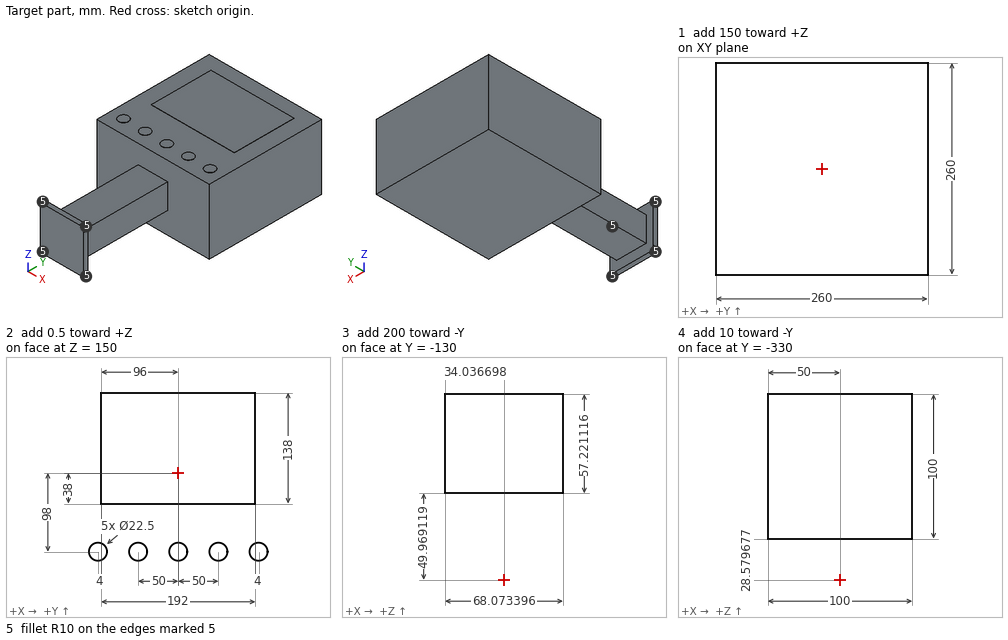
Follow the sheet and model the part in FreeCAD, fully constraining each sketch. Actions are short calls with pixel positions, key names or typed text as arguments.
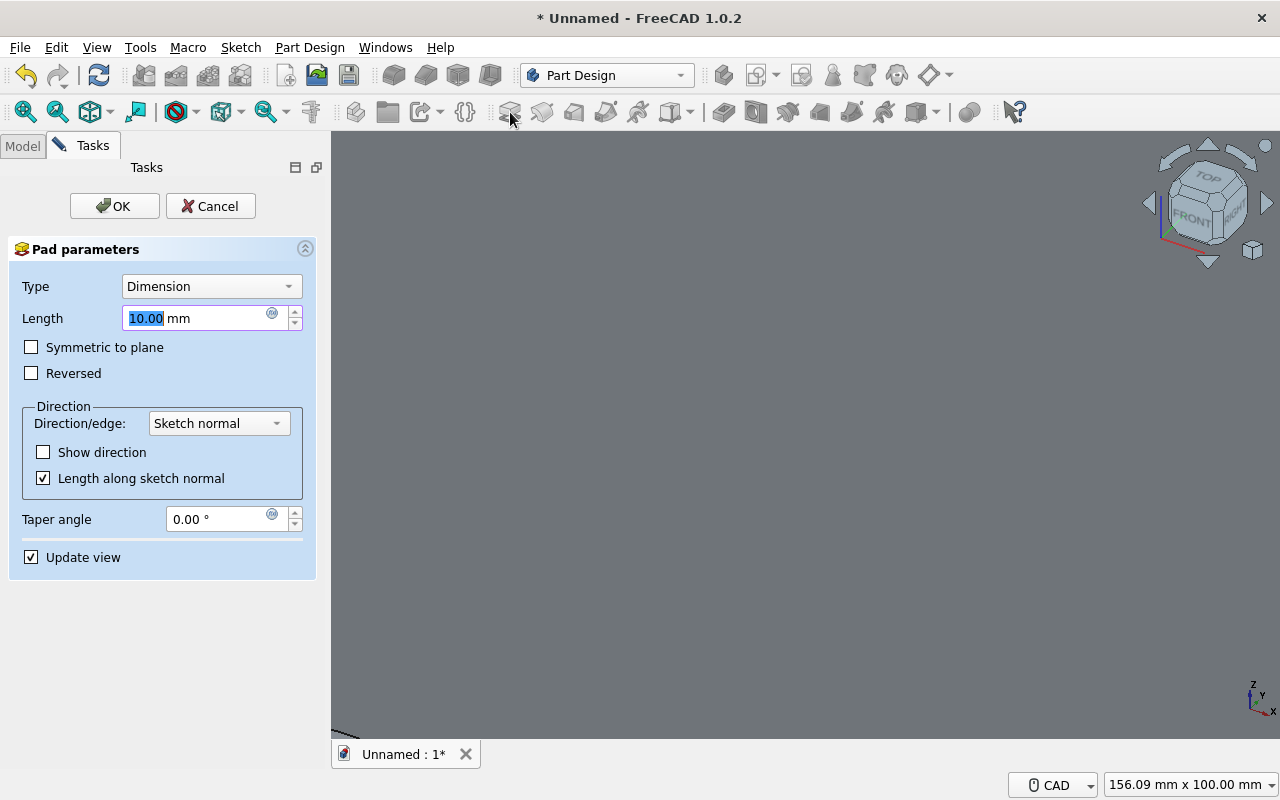
text(150)
key(Tab)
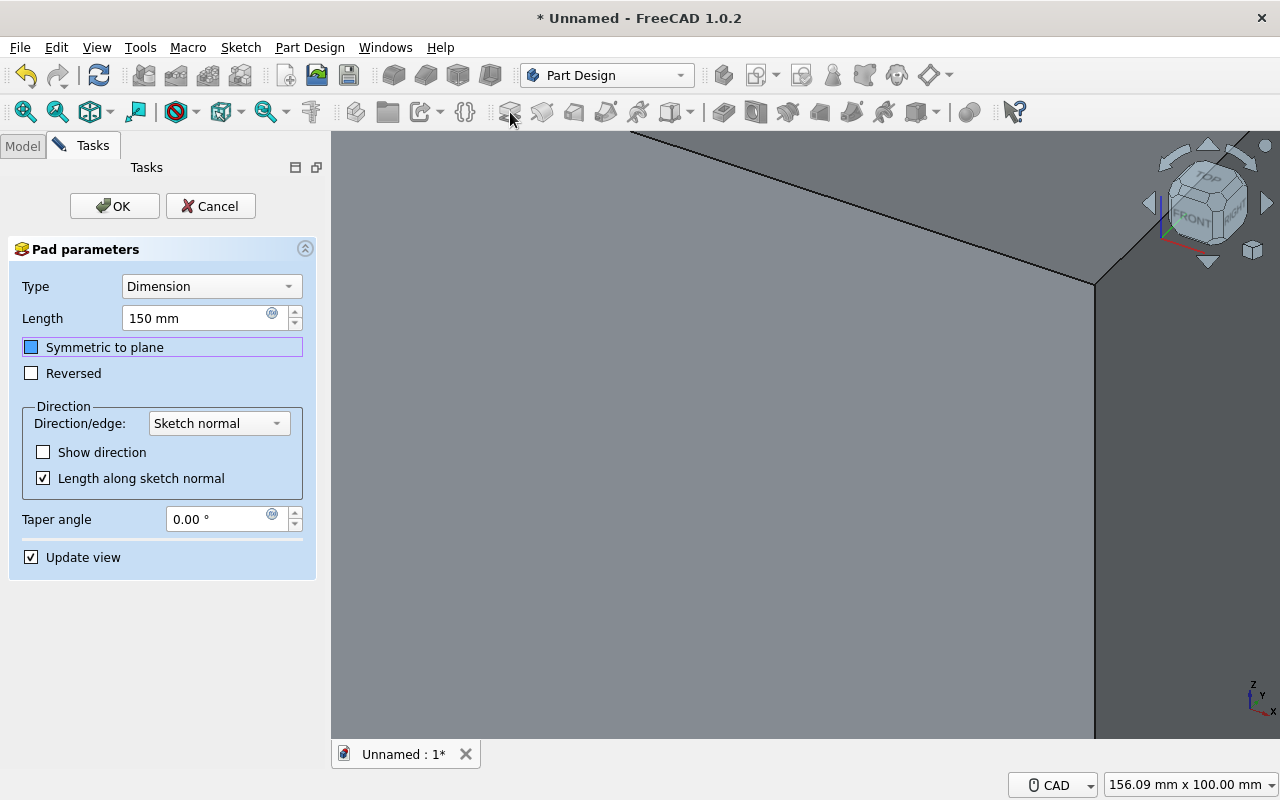
click(115, 206)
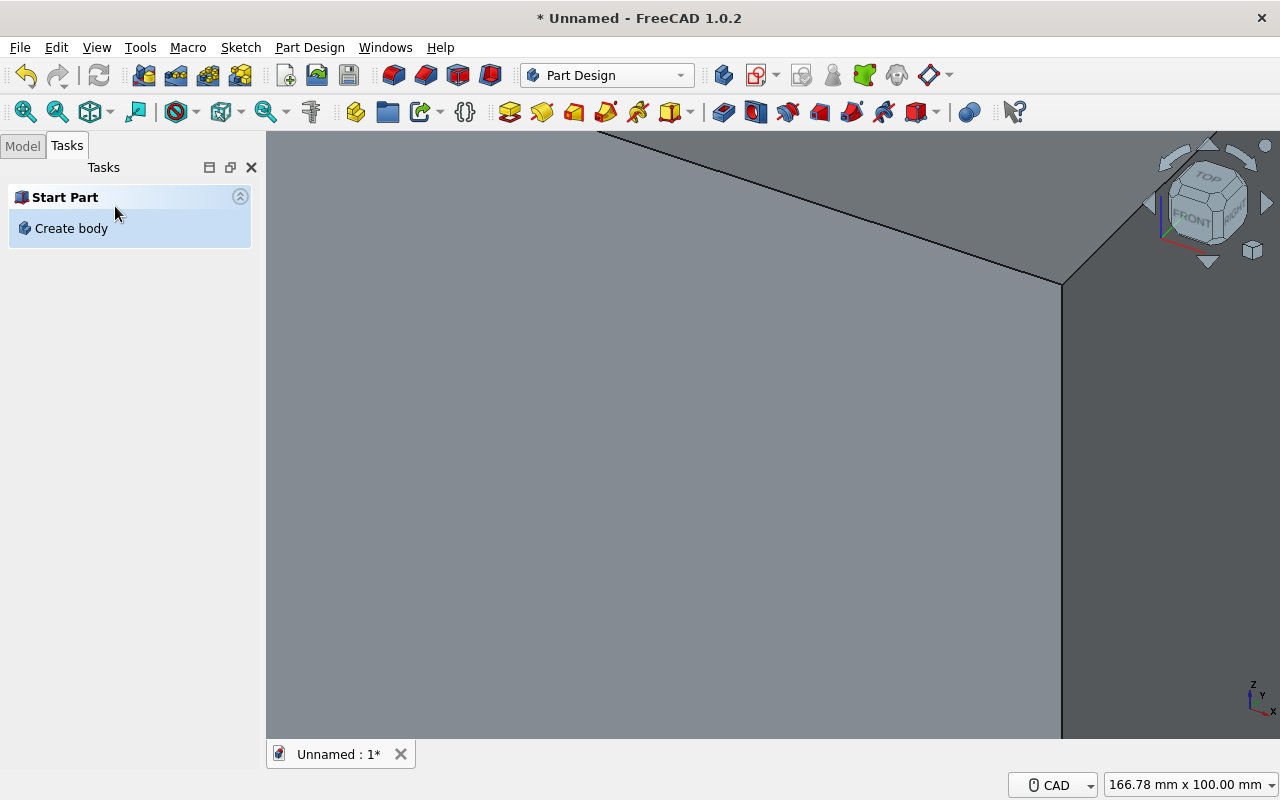
key(v)
key(f)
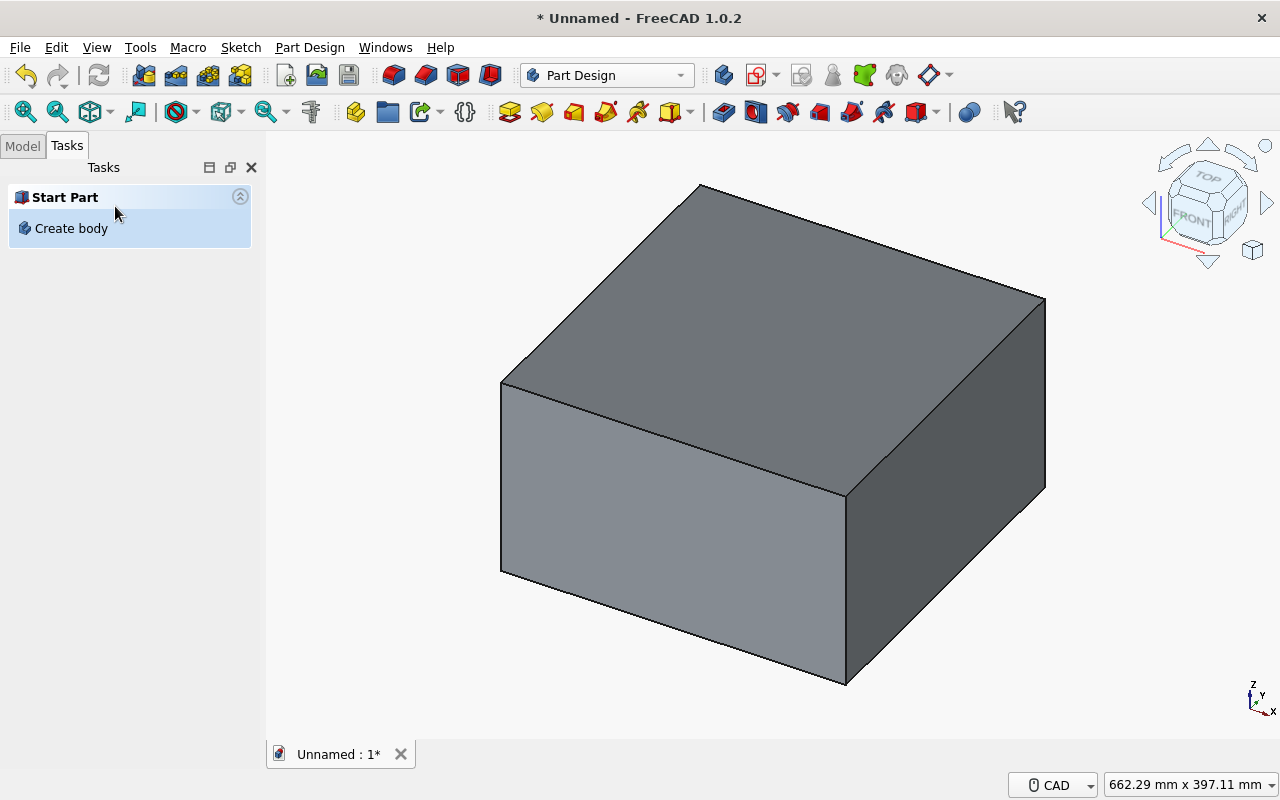
click(773, 340)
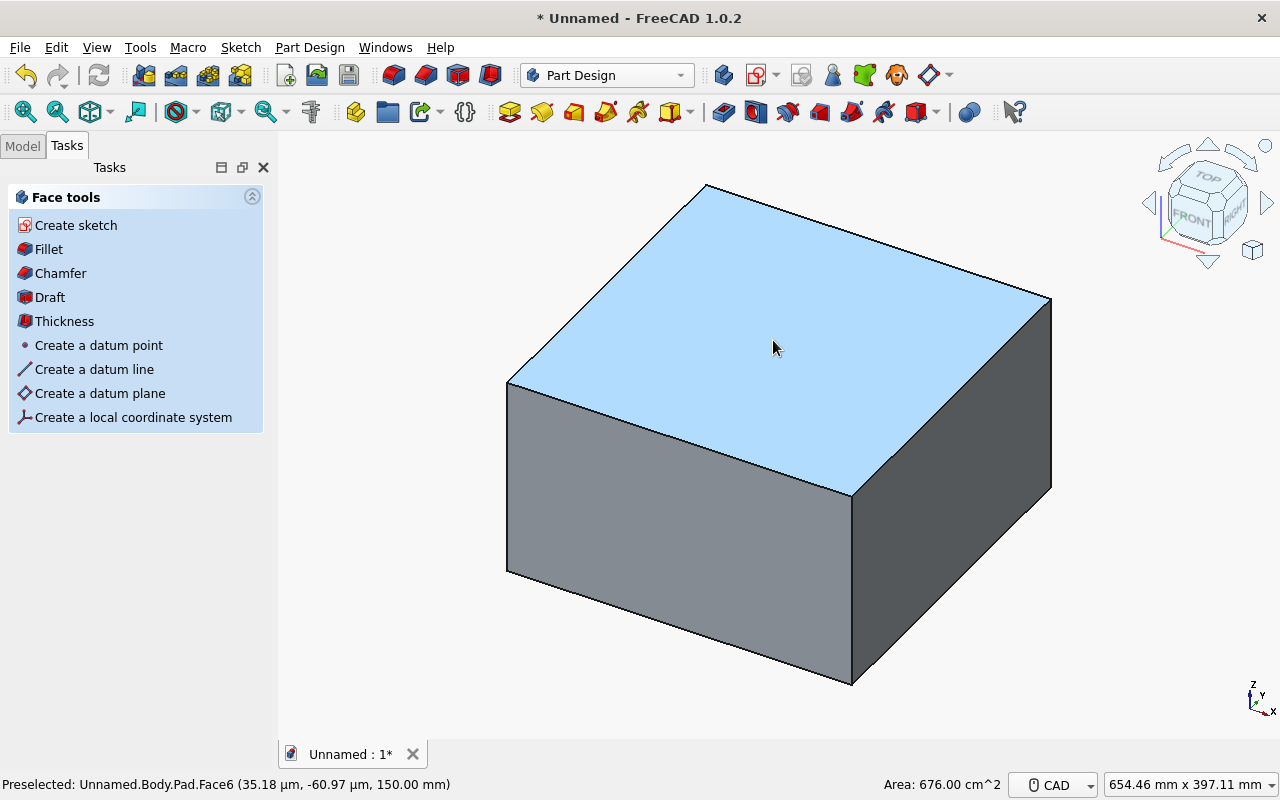
click(756, 76)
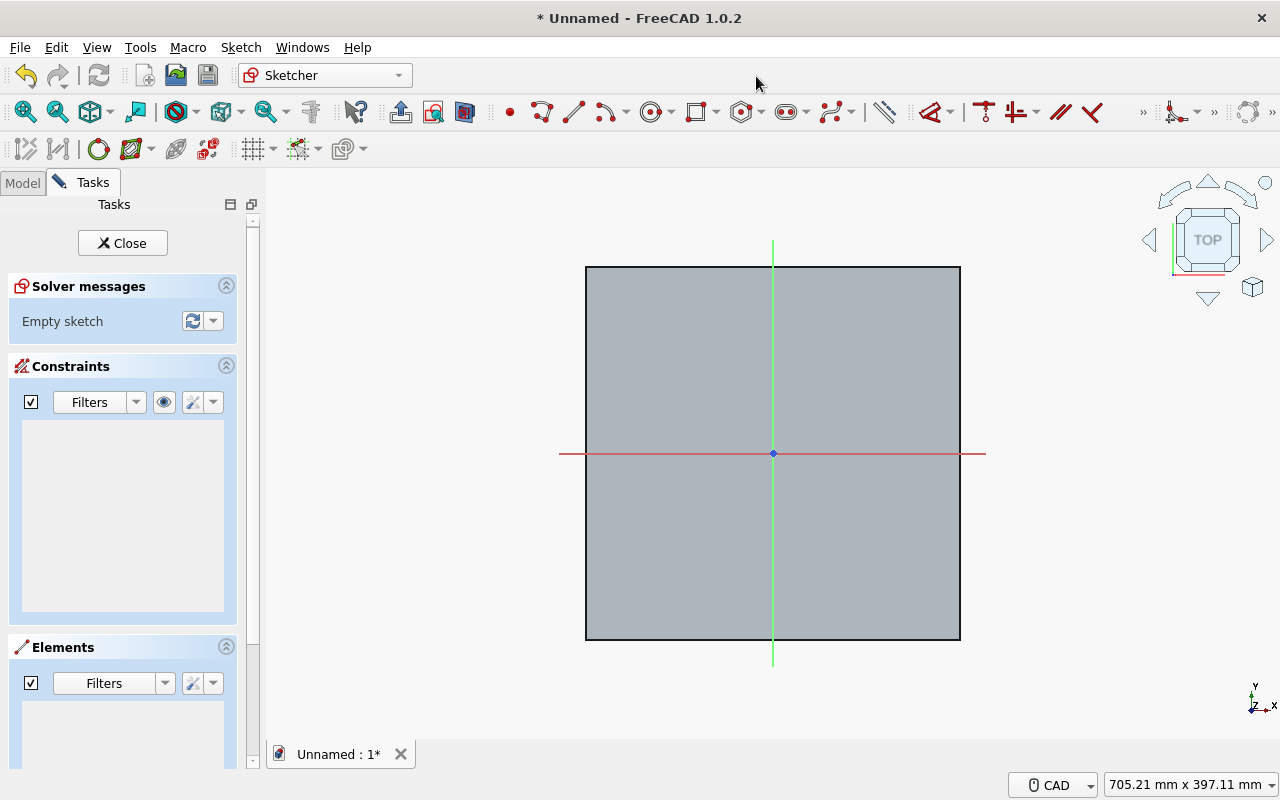
click(696, 112)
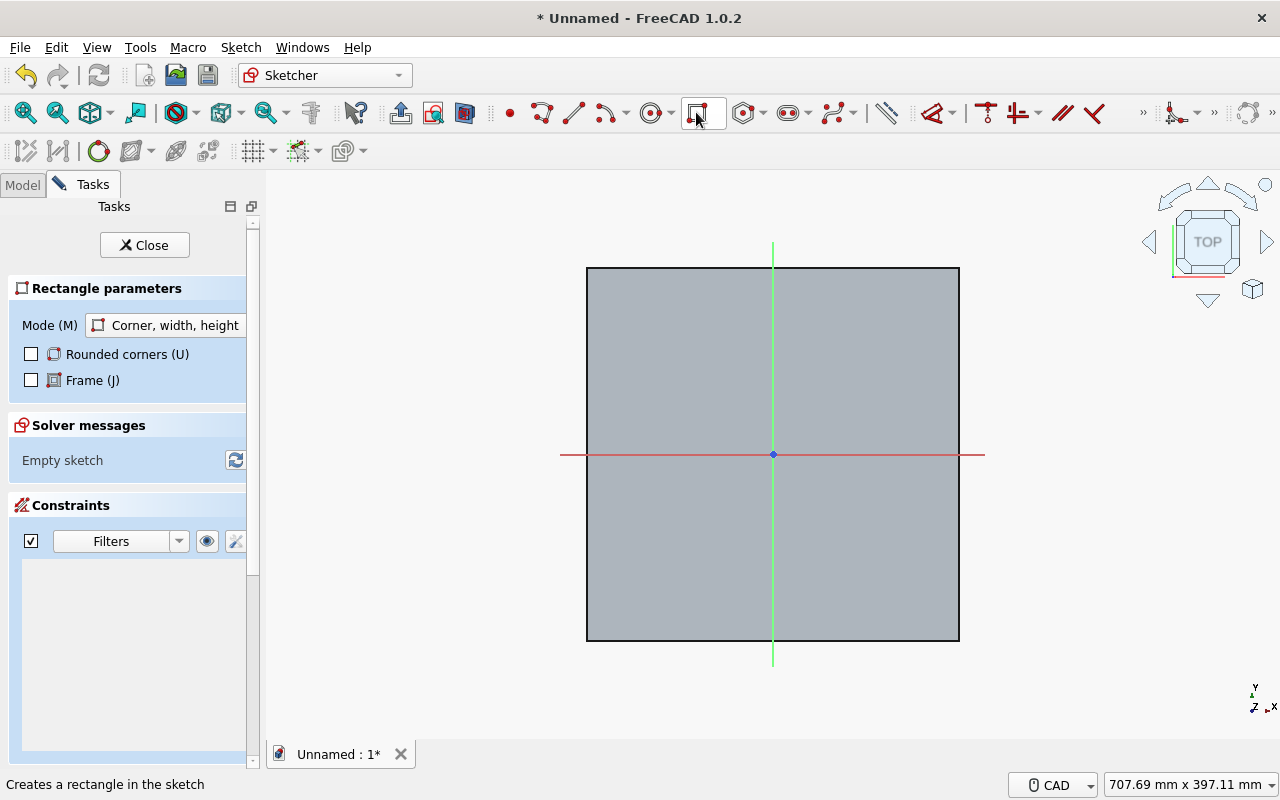
click(635, 311)
move(911, 509)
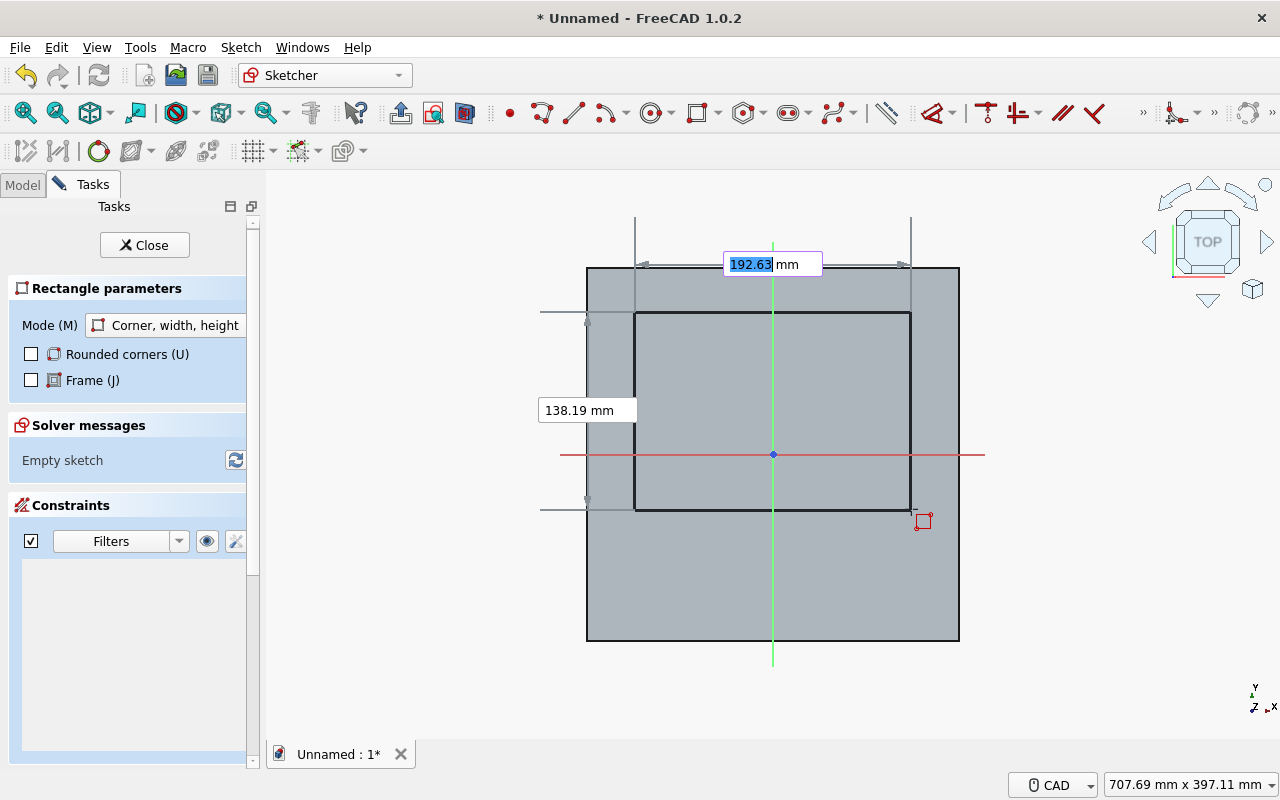
text(192)
key(Tab)
text(138)
key(Return)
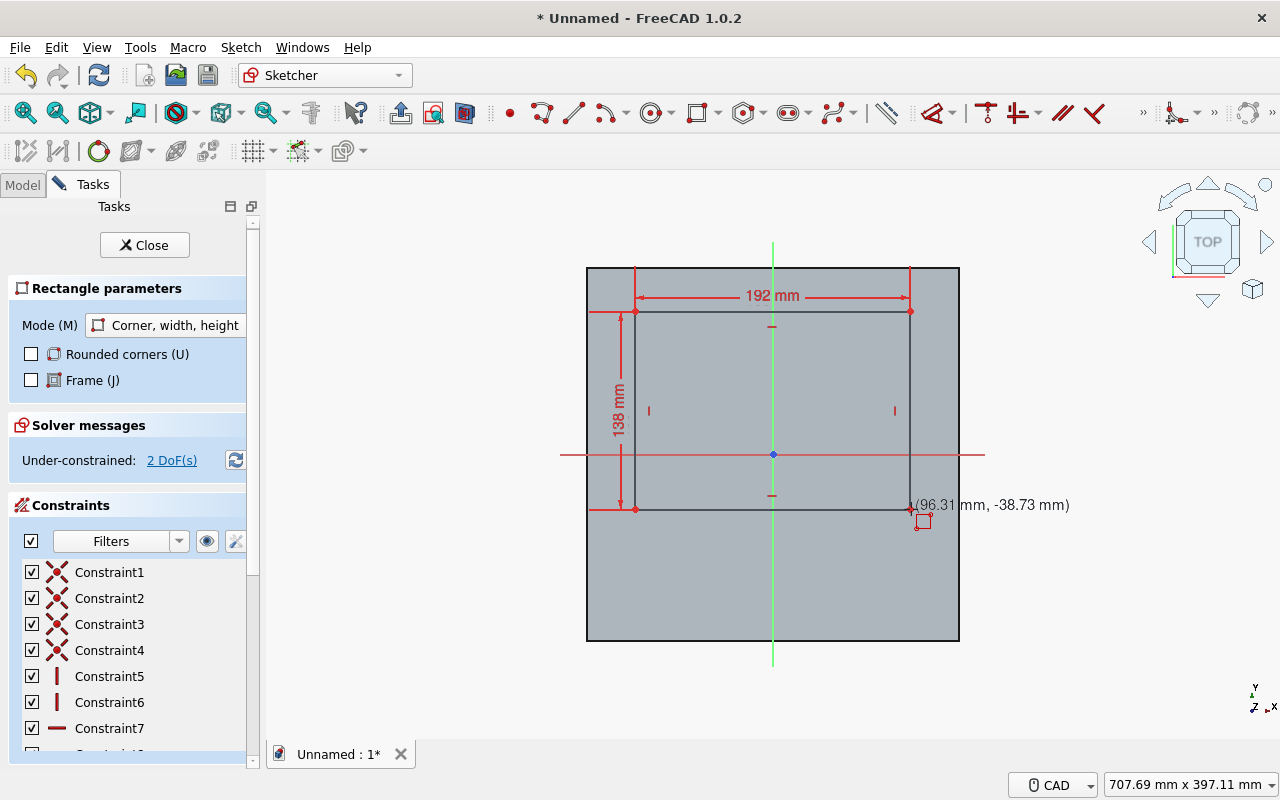
key(g)
key(c)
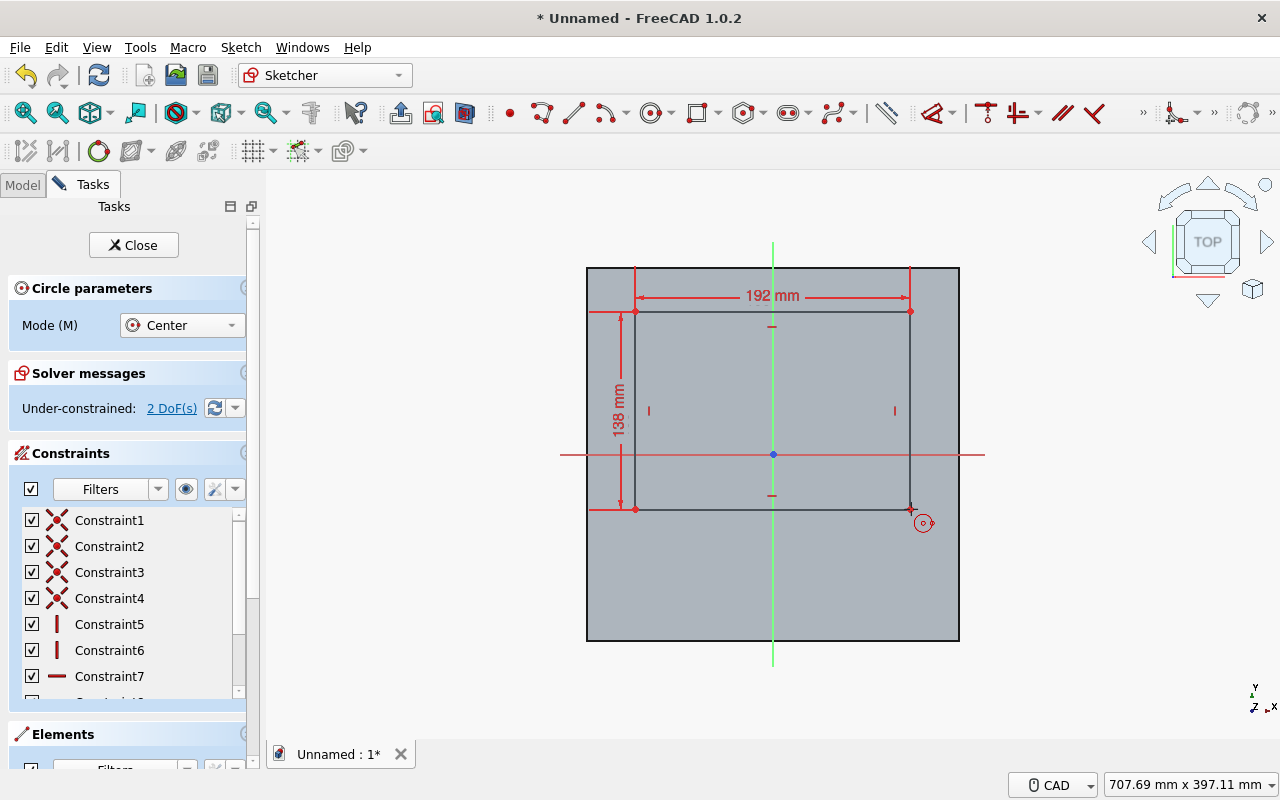
scroll(630, 595, up, 2)